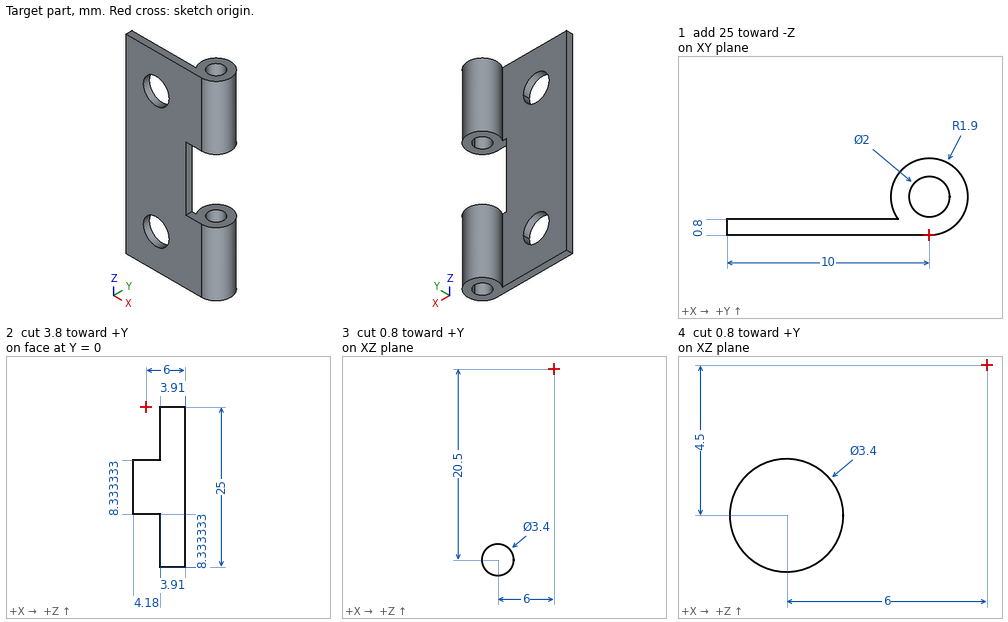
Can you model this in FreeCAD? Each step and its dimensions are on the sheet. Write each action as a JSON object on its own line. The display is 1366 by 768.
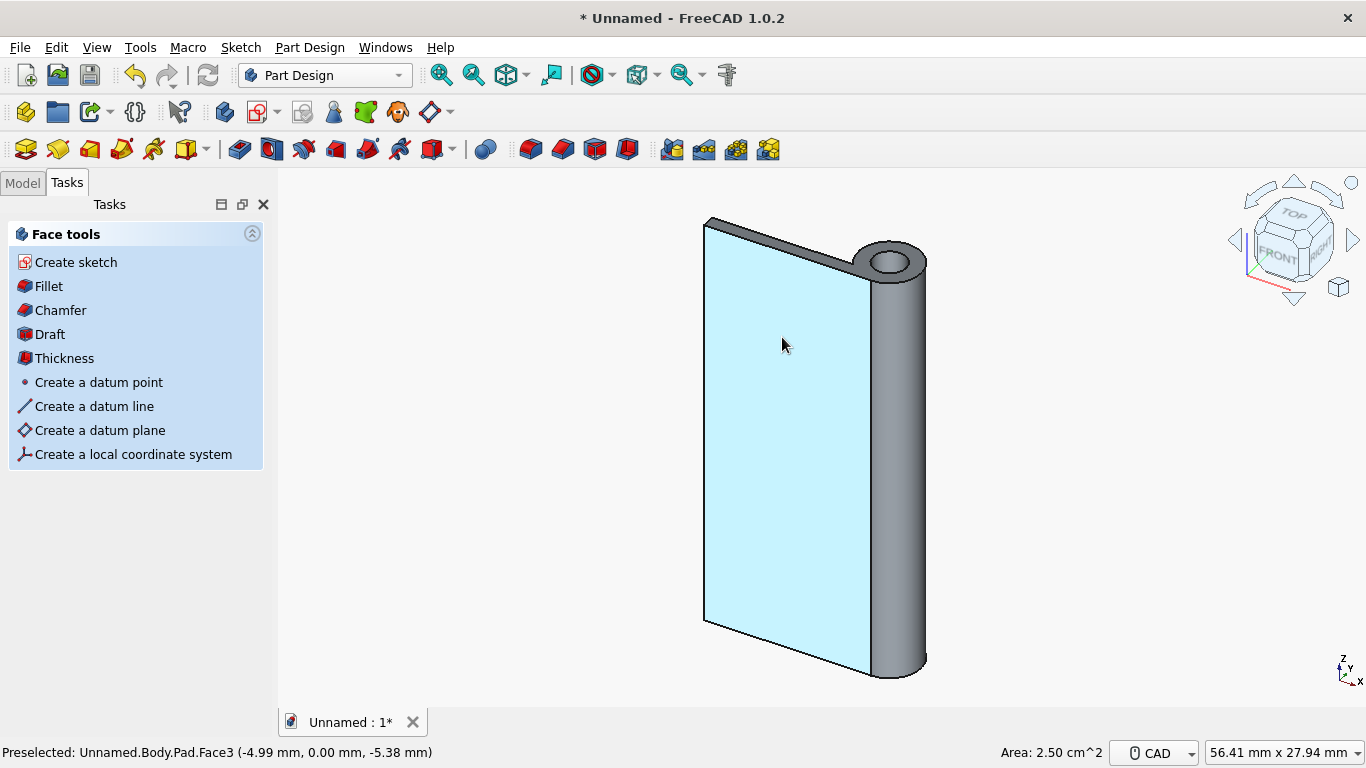
{"action": "left_click", "coordinate": [258, 112]}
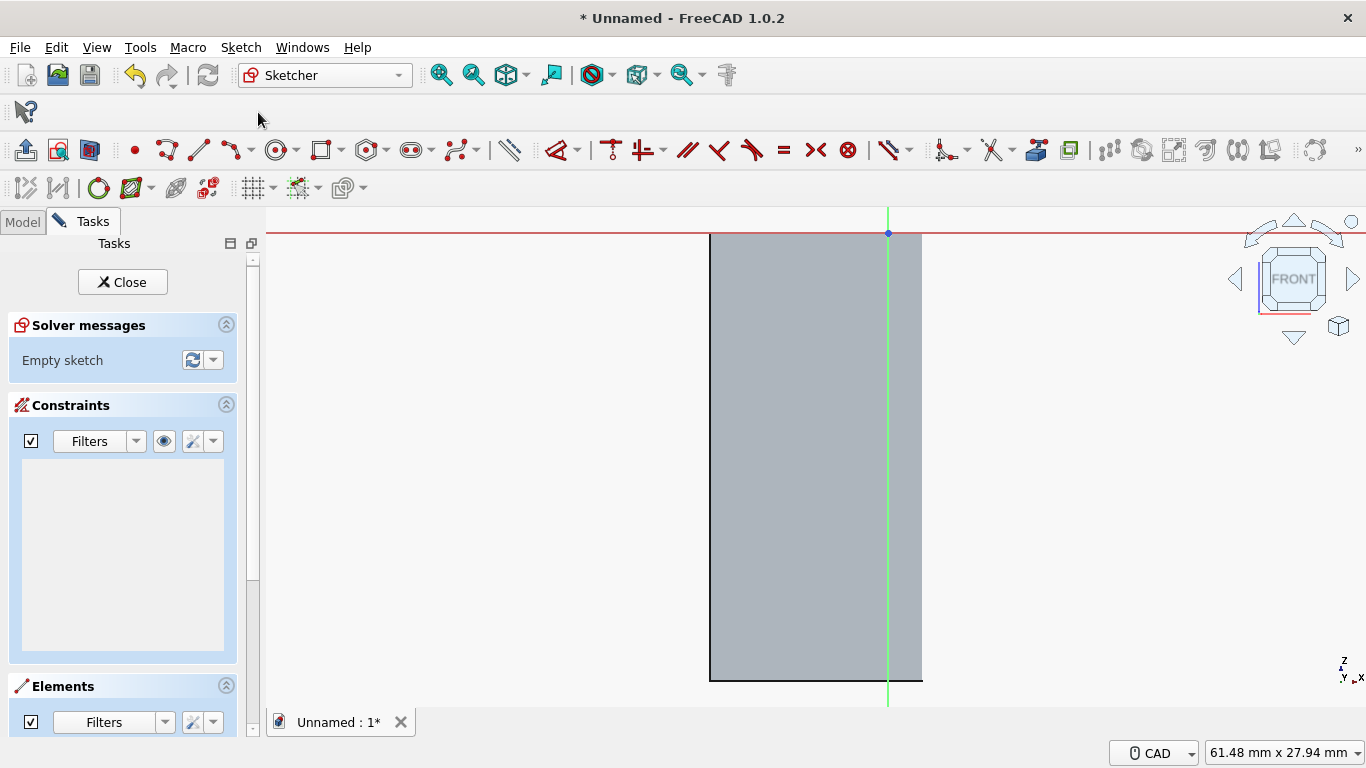
{"action": "scroll", "coordinate": [390, 457], "scroll_direction": "down", "scroll_amount": 2}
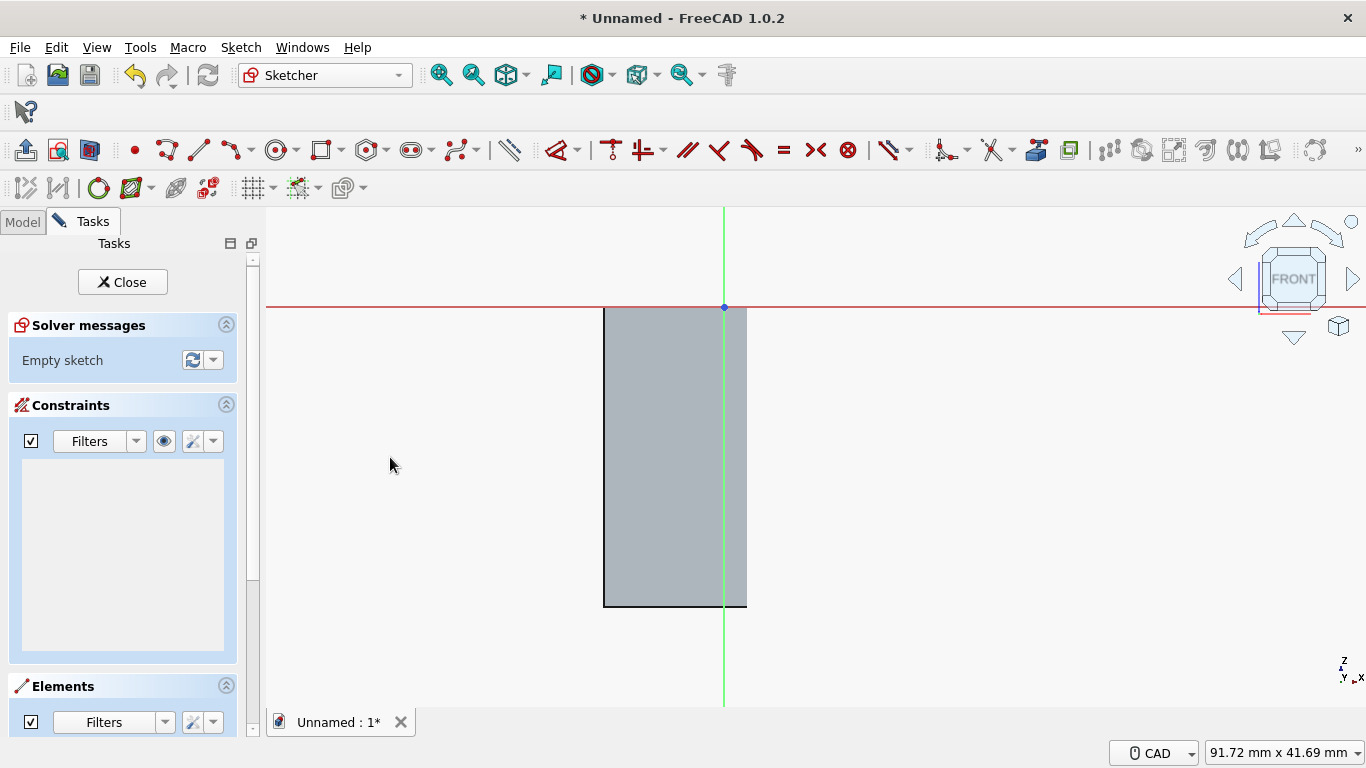
{"action": "left_click", "coordinate": [168, 150]}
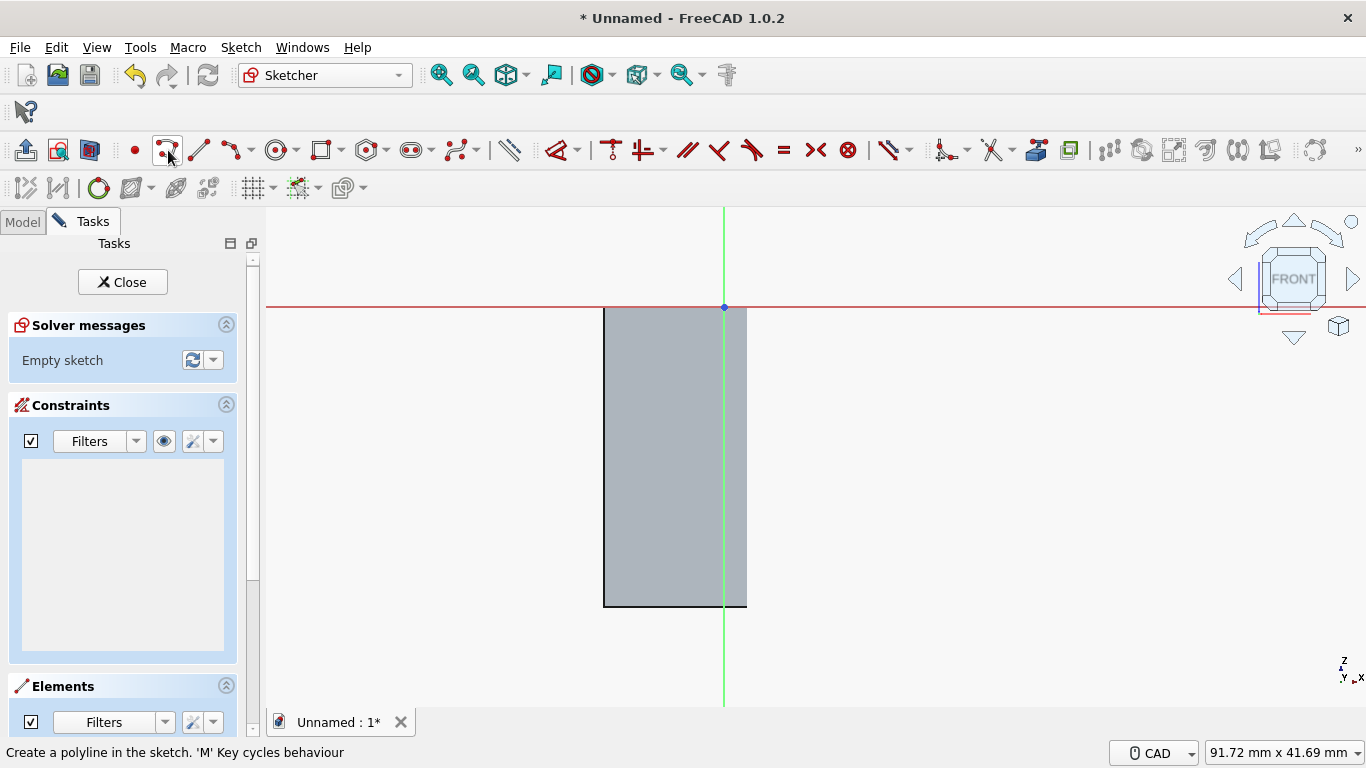
{"action": "left_click", "coordinate": [749, 307]}
{"action": "left_click", "coordinate": [796, 316]}
{"action": "left_click", "coordinate": [796, 607]}
{"action": "left_click", "coordinate": [749, 607]}
{"action": "left_click", "coordinate": [749, 507]}
{"action": "left_click", "coordinate": [699, 507]}
{"action": "left_click", "coordinate": [699, 407]}
{"action": "left_click", "coordinate": [749, 407]}
{"action": "left_click", "coordinate": [749, 307]}
{"action": "key", "text": "Escape"}
{"action": "key", "text": "Escape"}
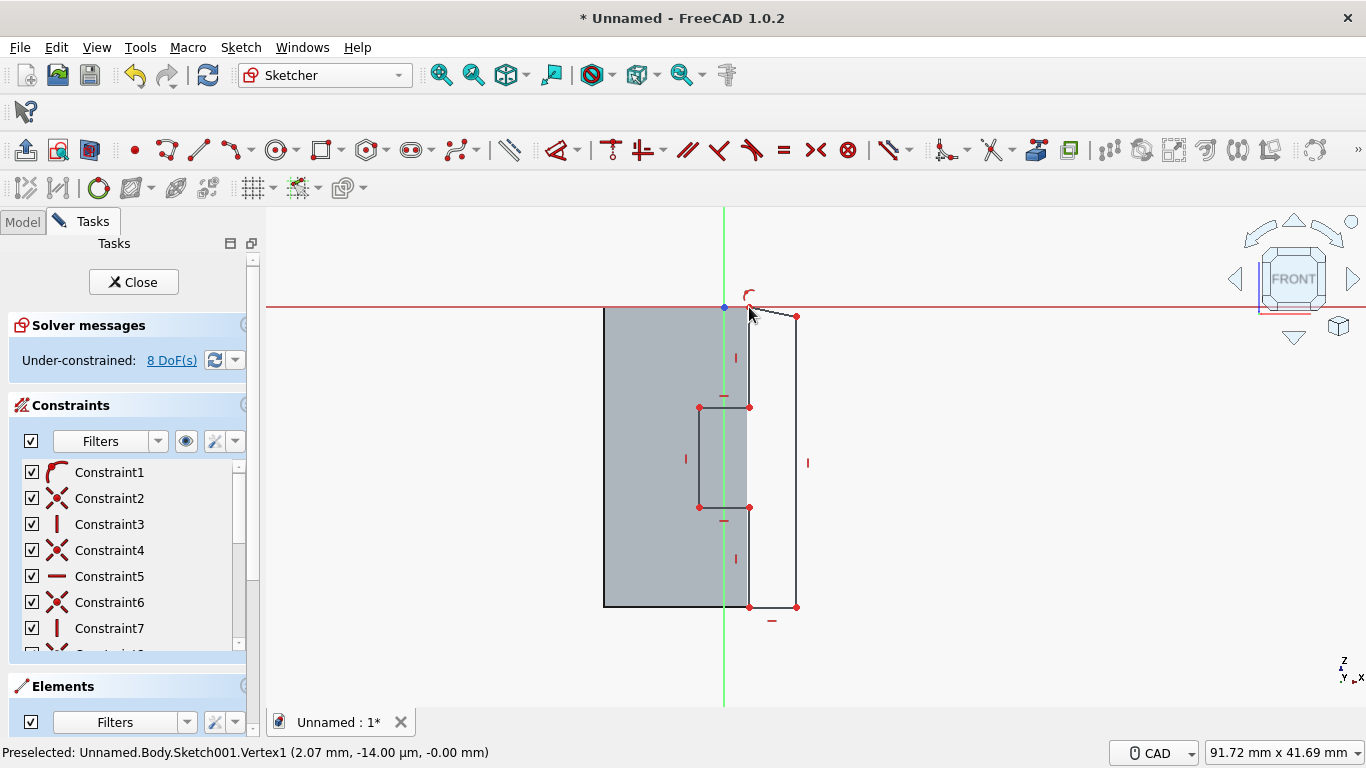
{"action": "left_click", "coordinate": [763, 310]}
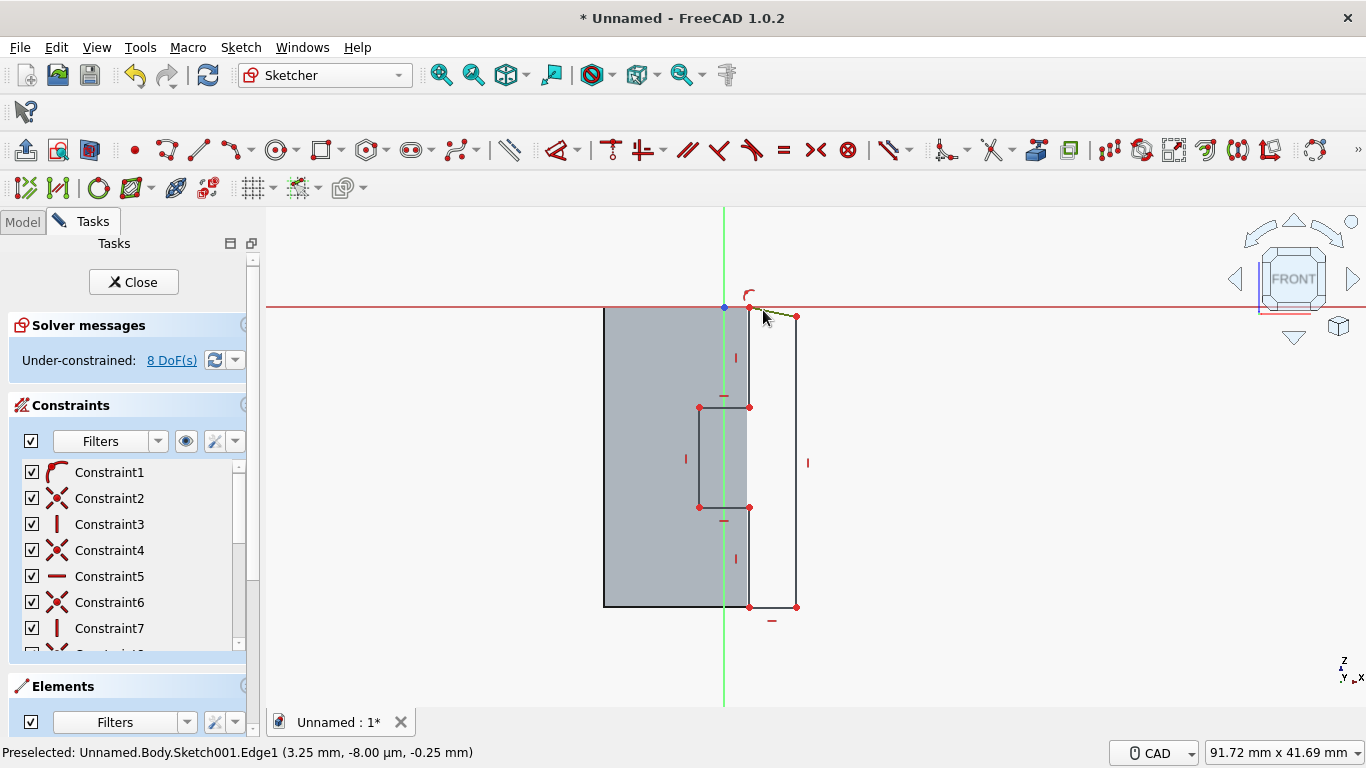
{"action": "key", "text": "h"}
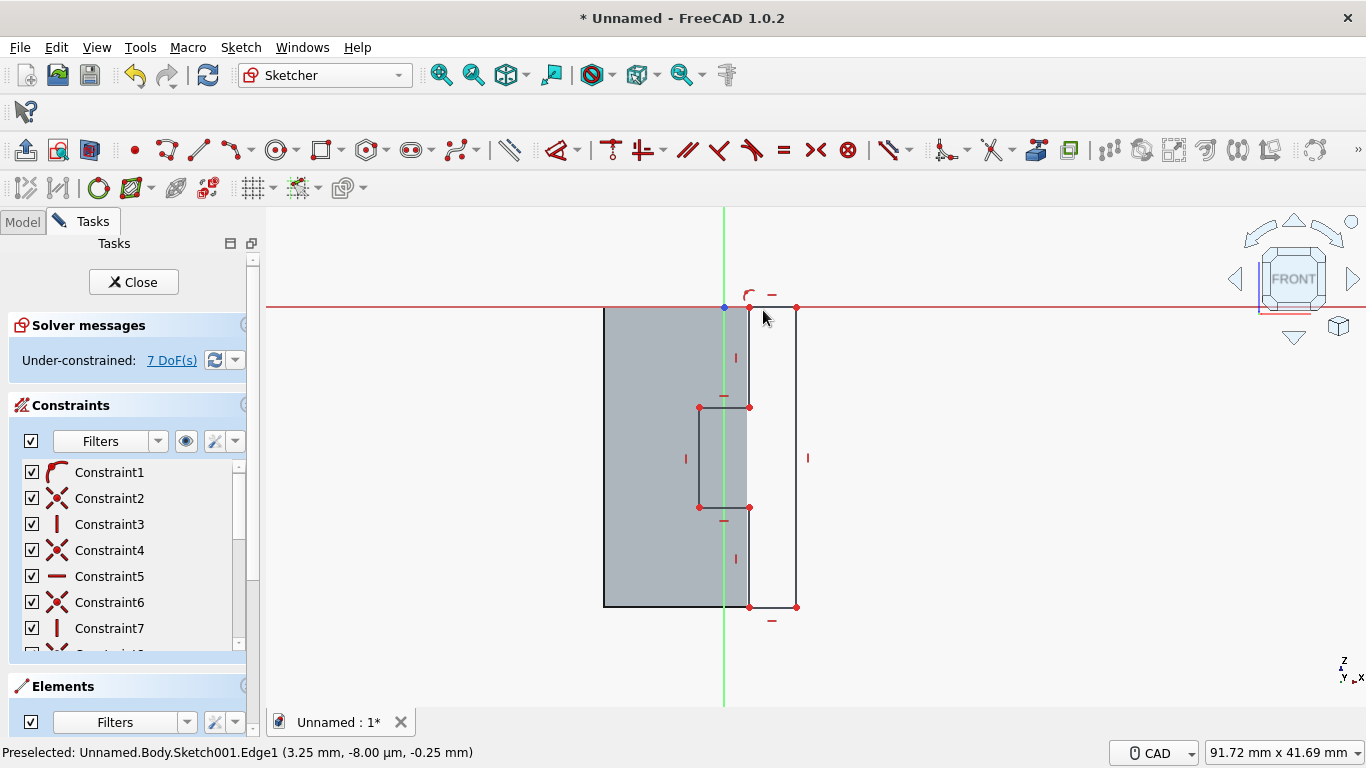
{"action": "left_click", "coordinate": [556, 150]}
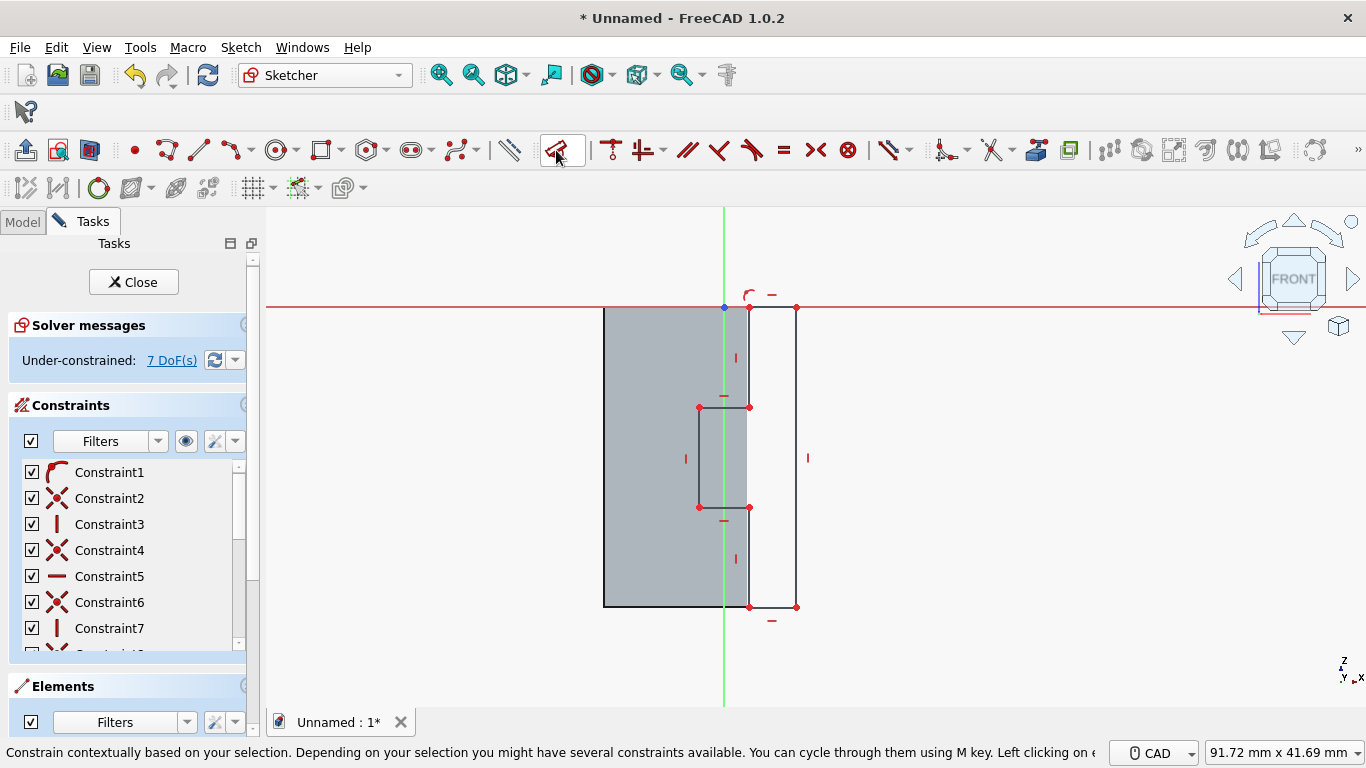
{"action": "left_click", "coordinate": [796, 397]}
{"action": "left_click", "coordinate": [830, 458]}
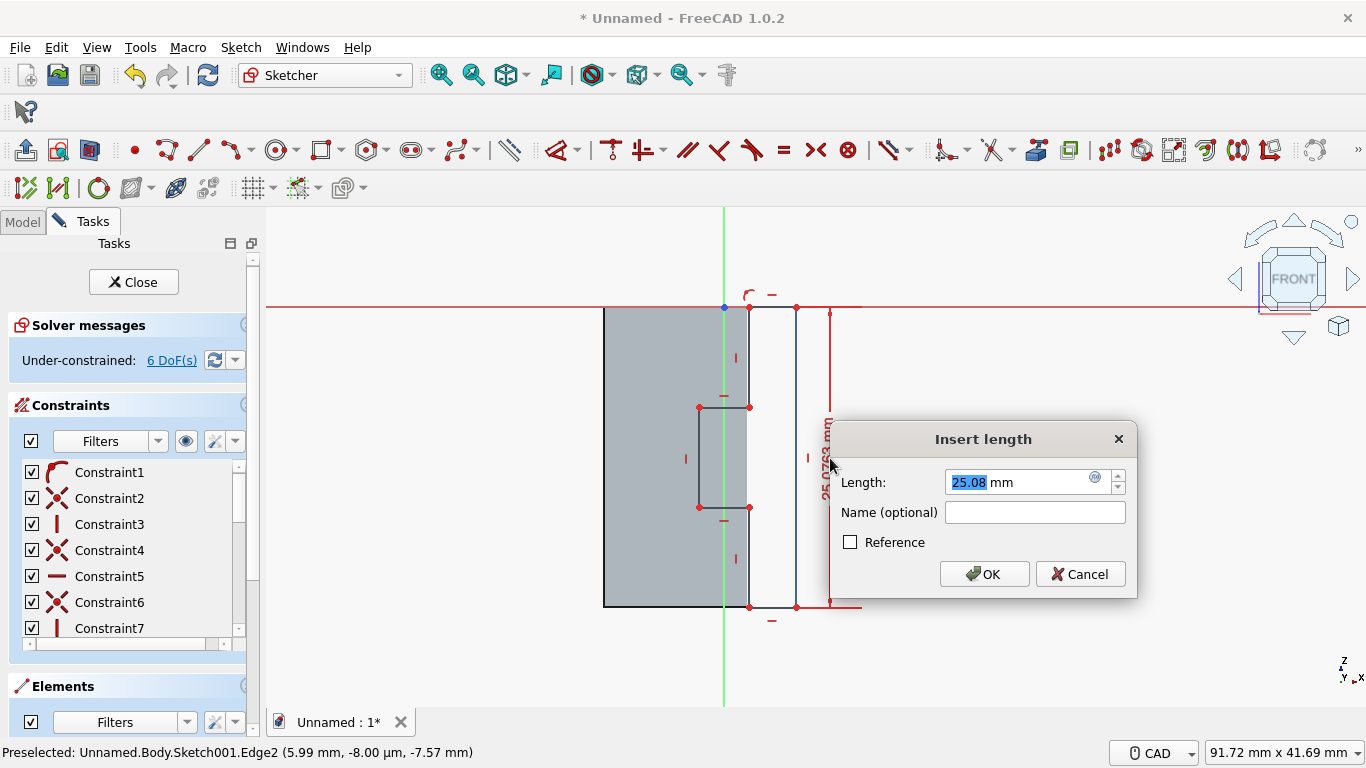
{"action": "type", "text": "25"}
{"action": "key", "text": "Return"}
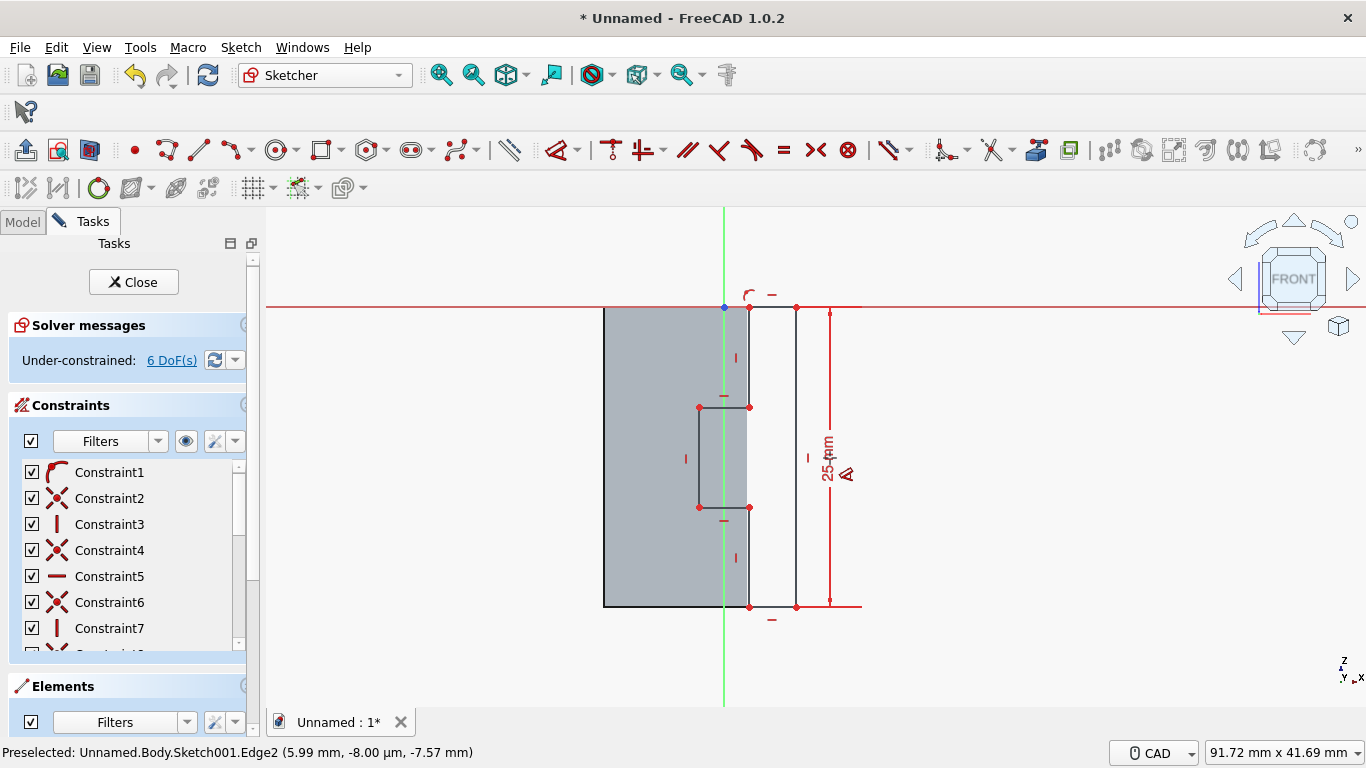
{"action": "left_click", "coordinate": [796, 307]}
{"action": "left_click", "coordinate": [760, 273]}